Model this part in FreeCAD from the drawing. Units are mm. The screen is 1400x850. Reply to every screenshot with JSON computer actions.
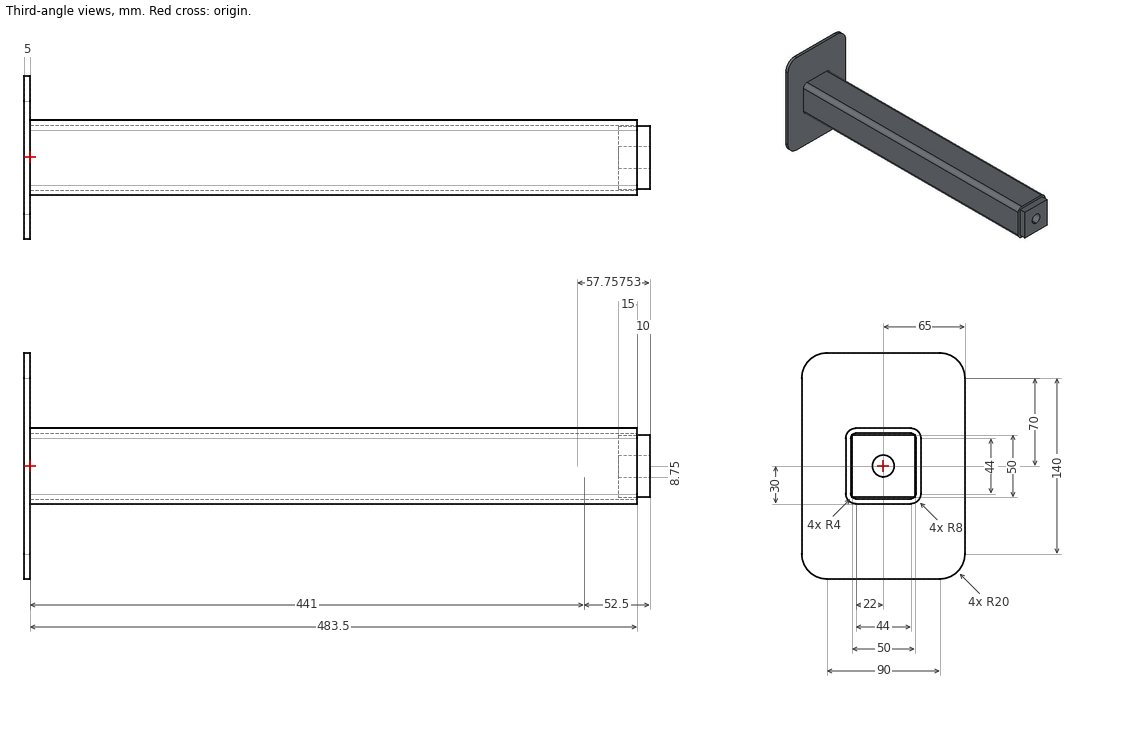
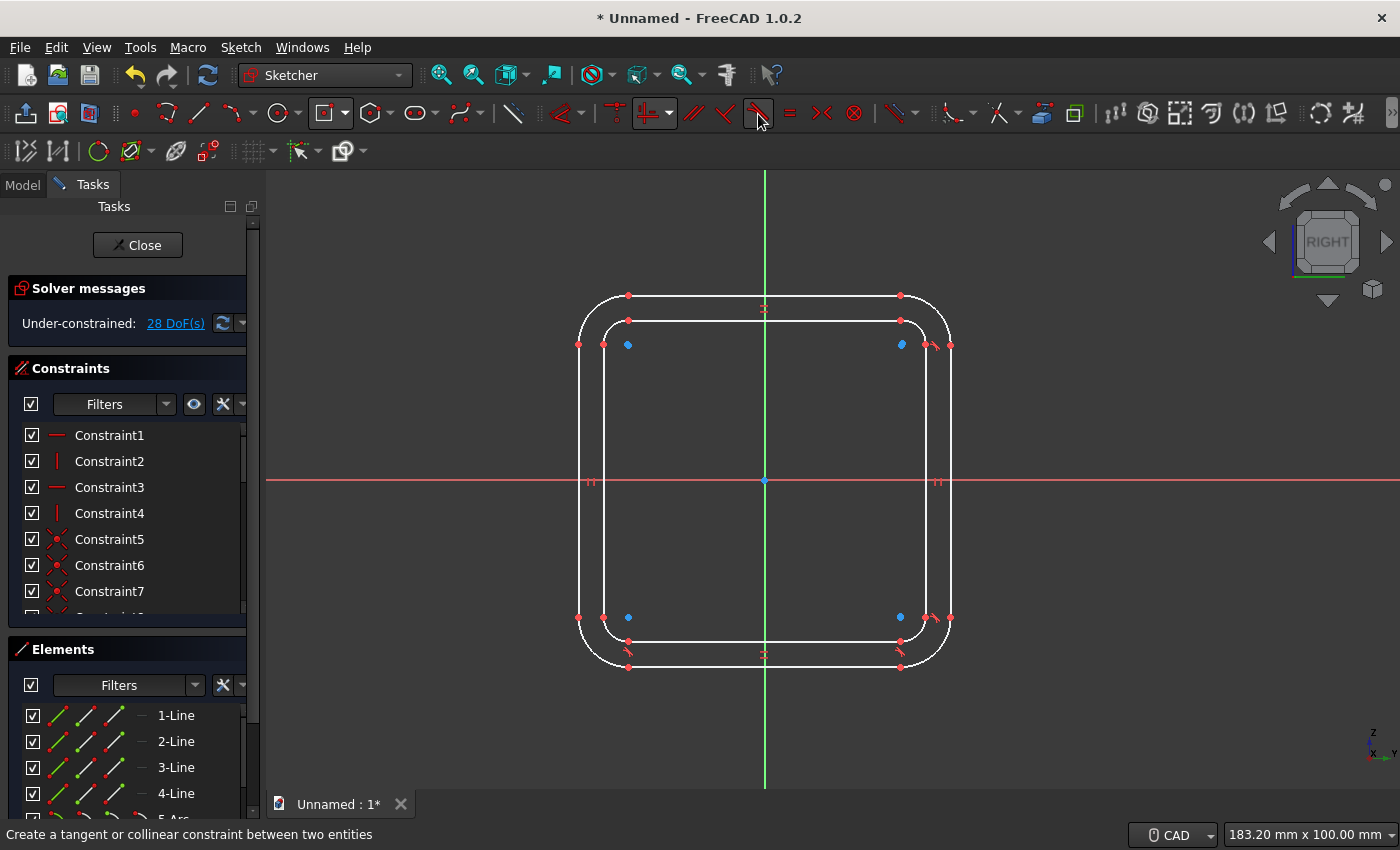
{"action": "left_click", "coordinate": [819, 296]}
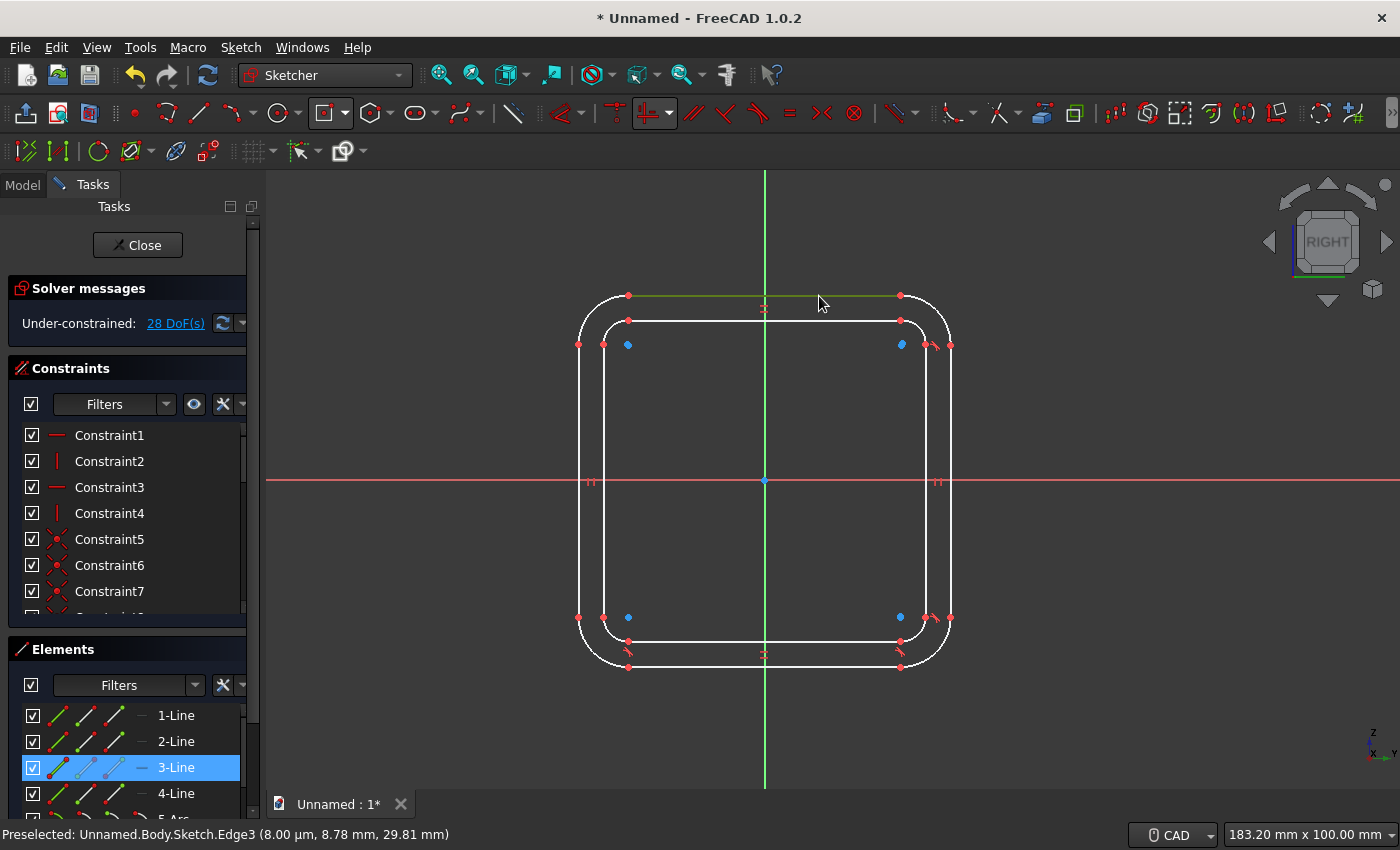
{"action": "left_click", "coordinate": [945, 322]}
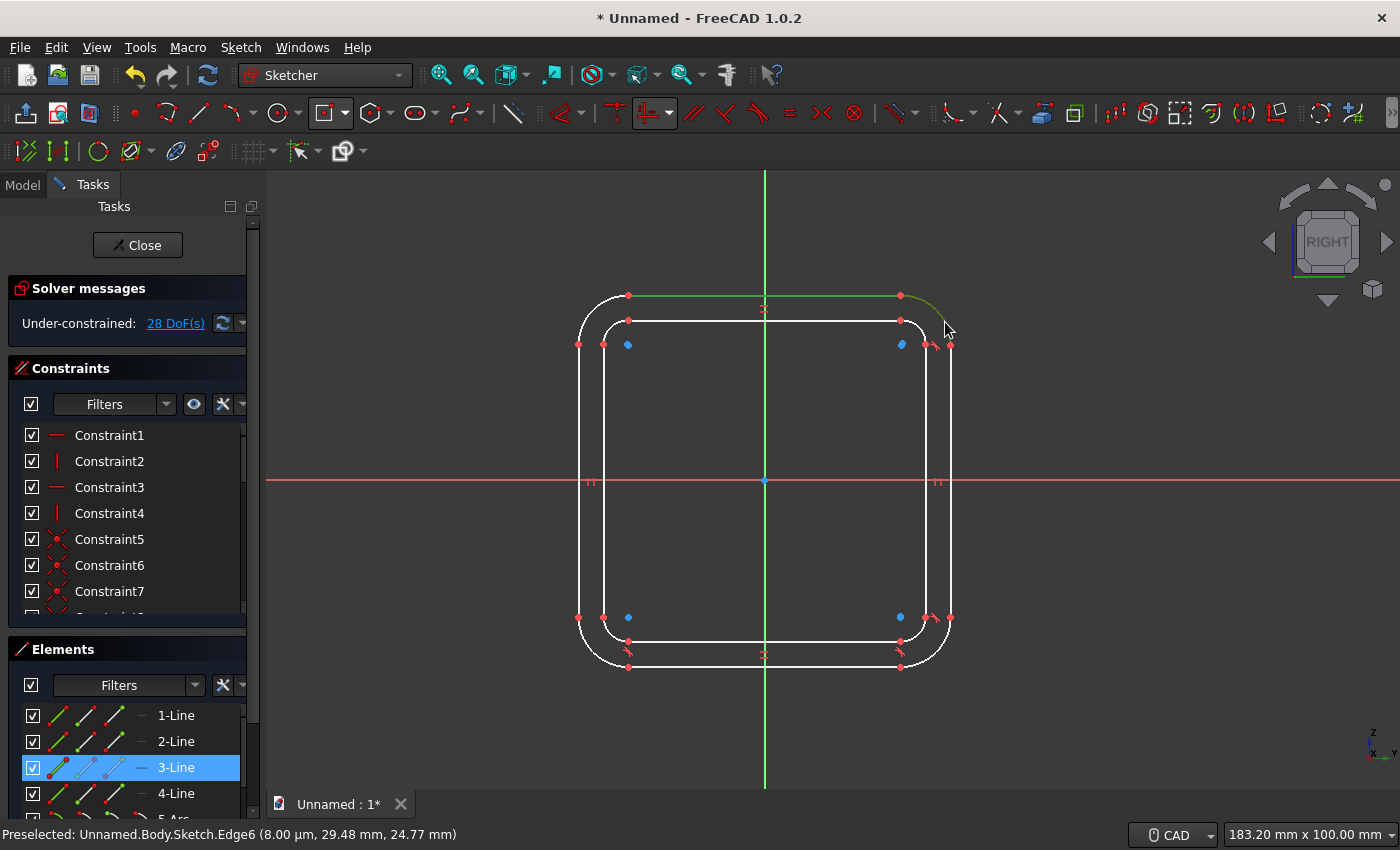
{"action": "key", "text": "t"}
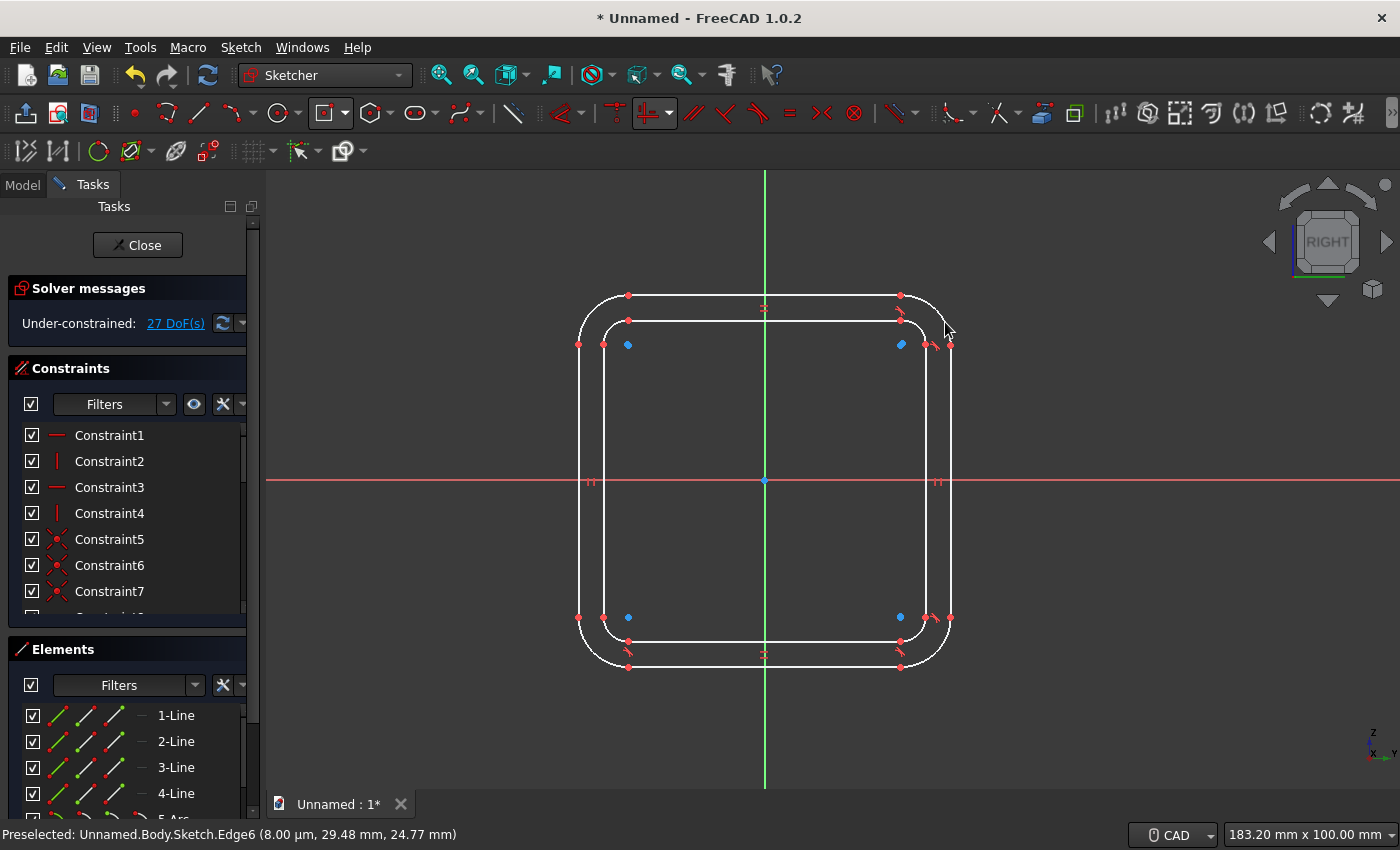
{"action": "left_click", "coordinate": [819, 295]}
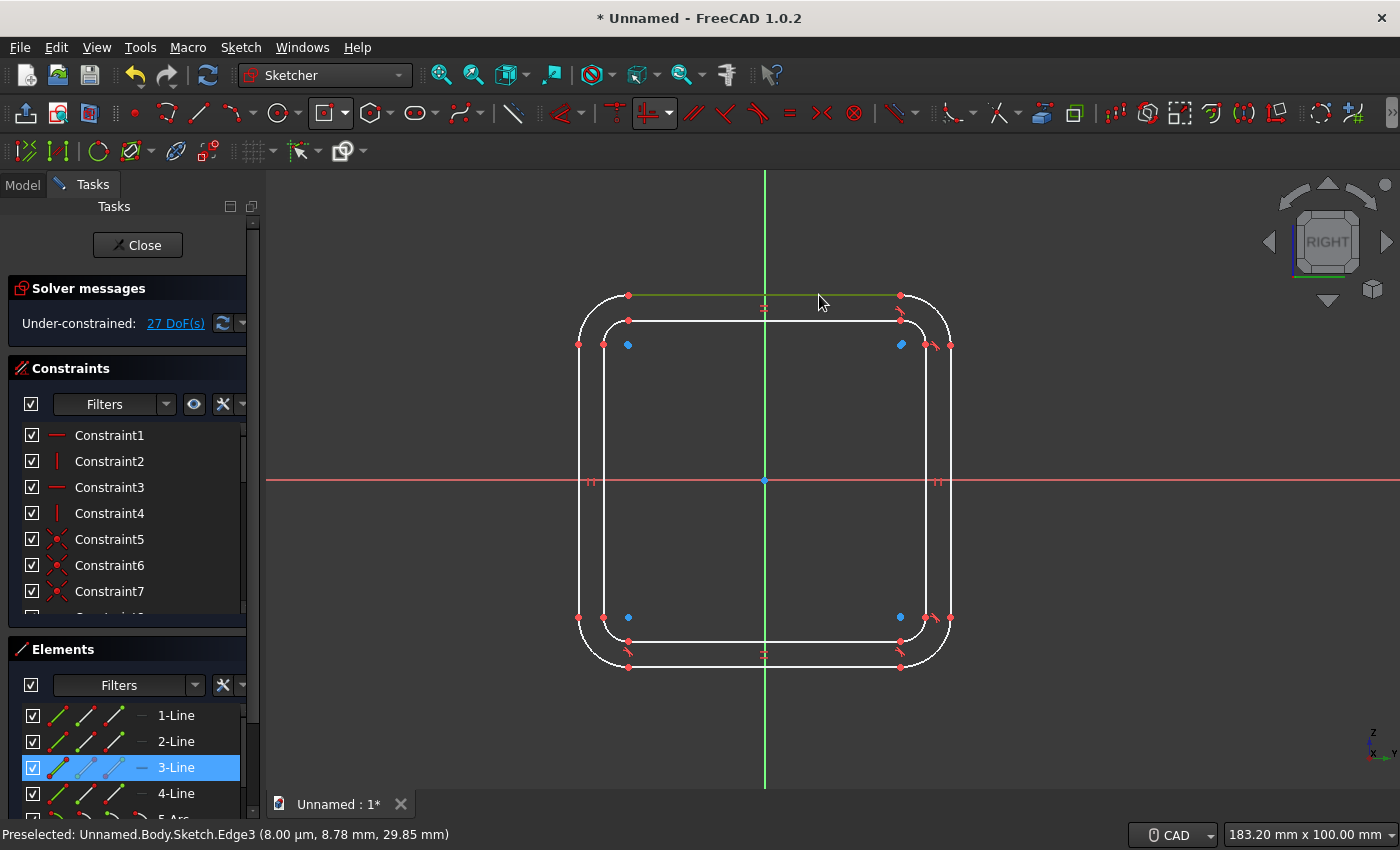
{"action": "left_click", "coordinate": [606, 301]}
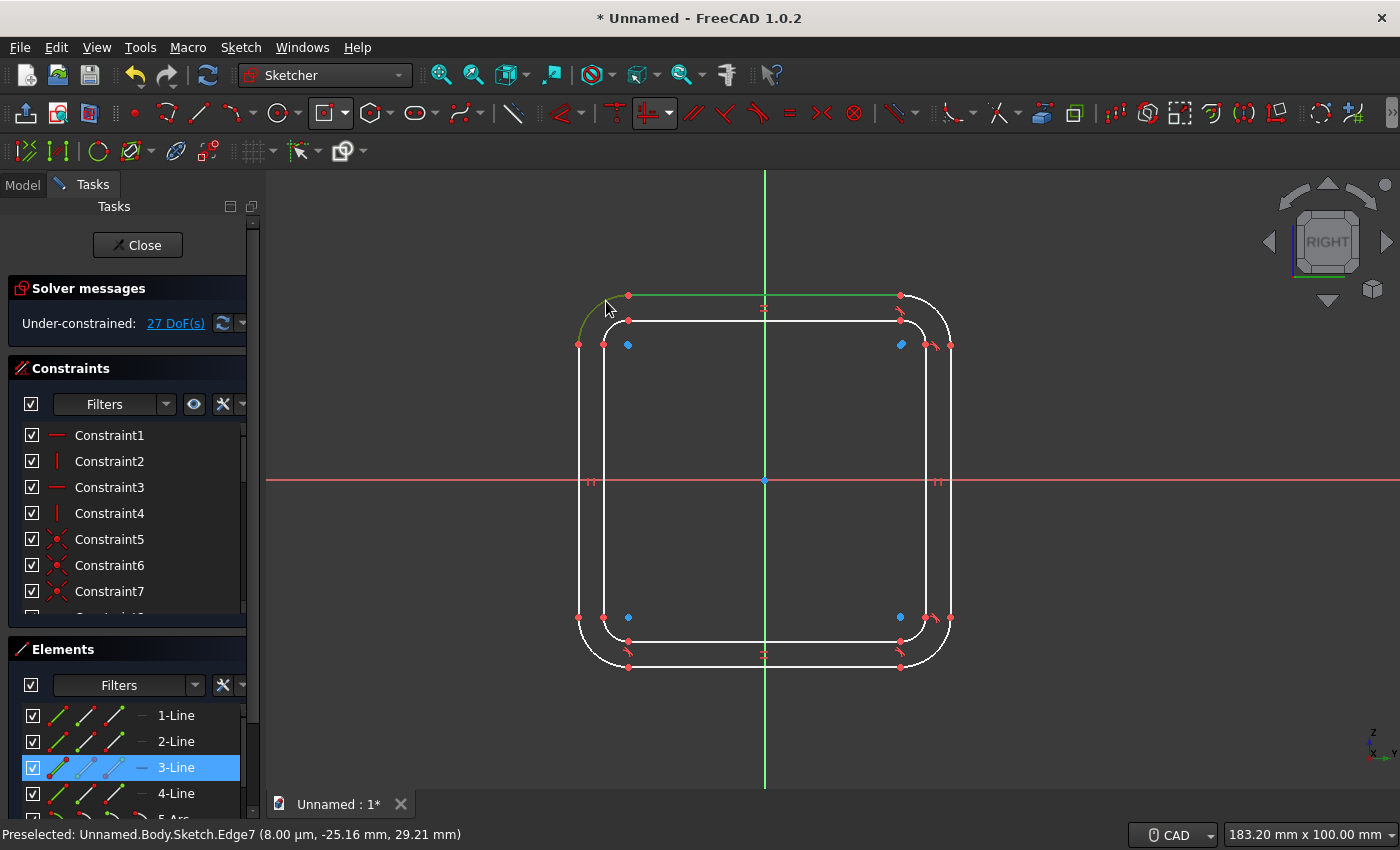
{"action": "left_click", "coordinate": [758, 114]}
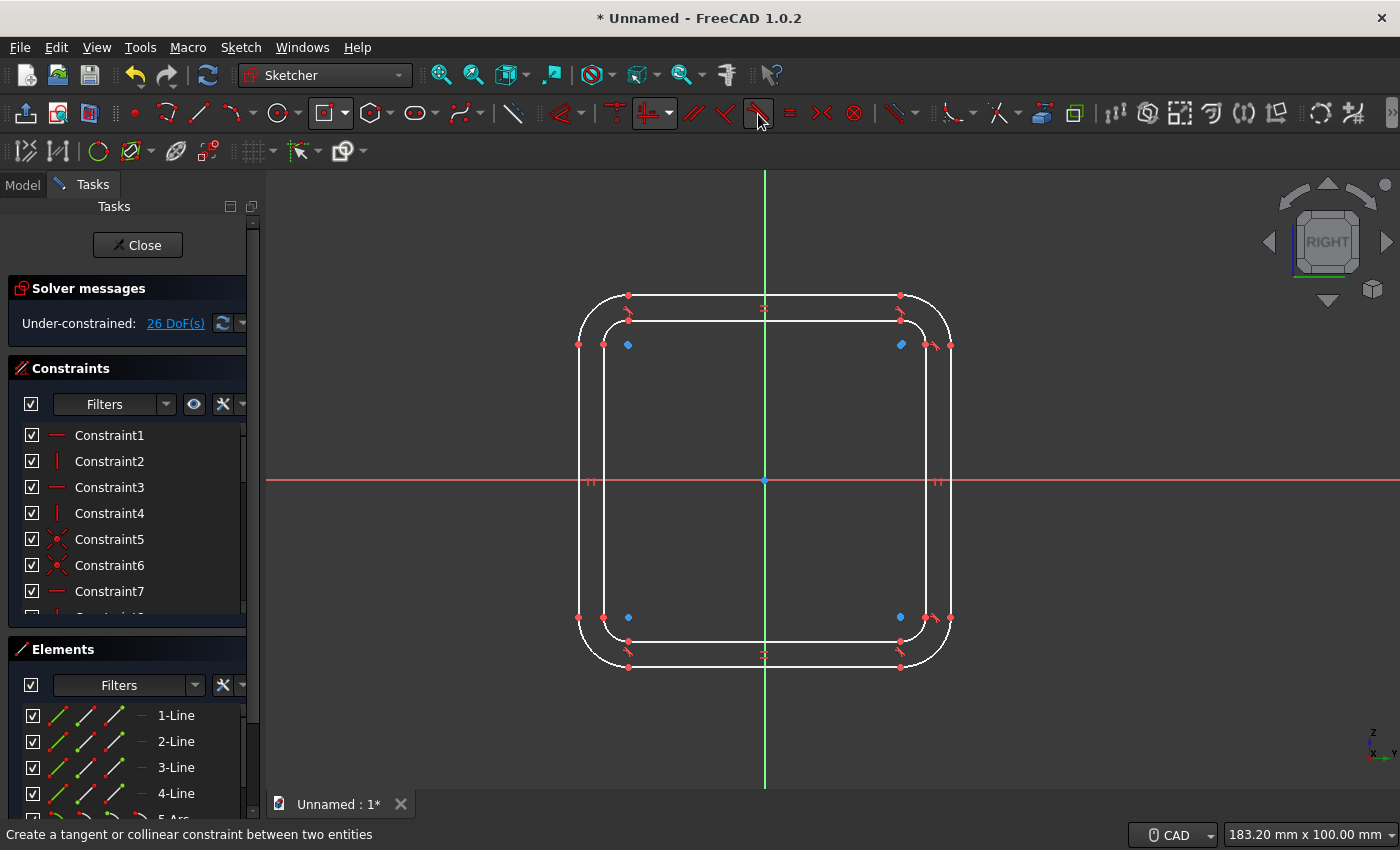
{"action": "left_click", "coordinate": [579, 426]}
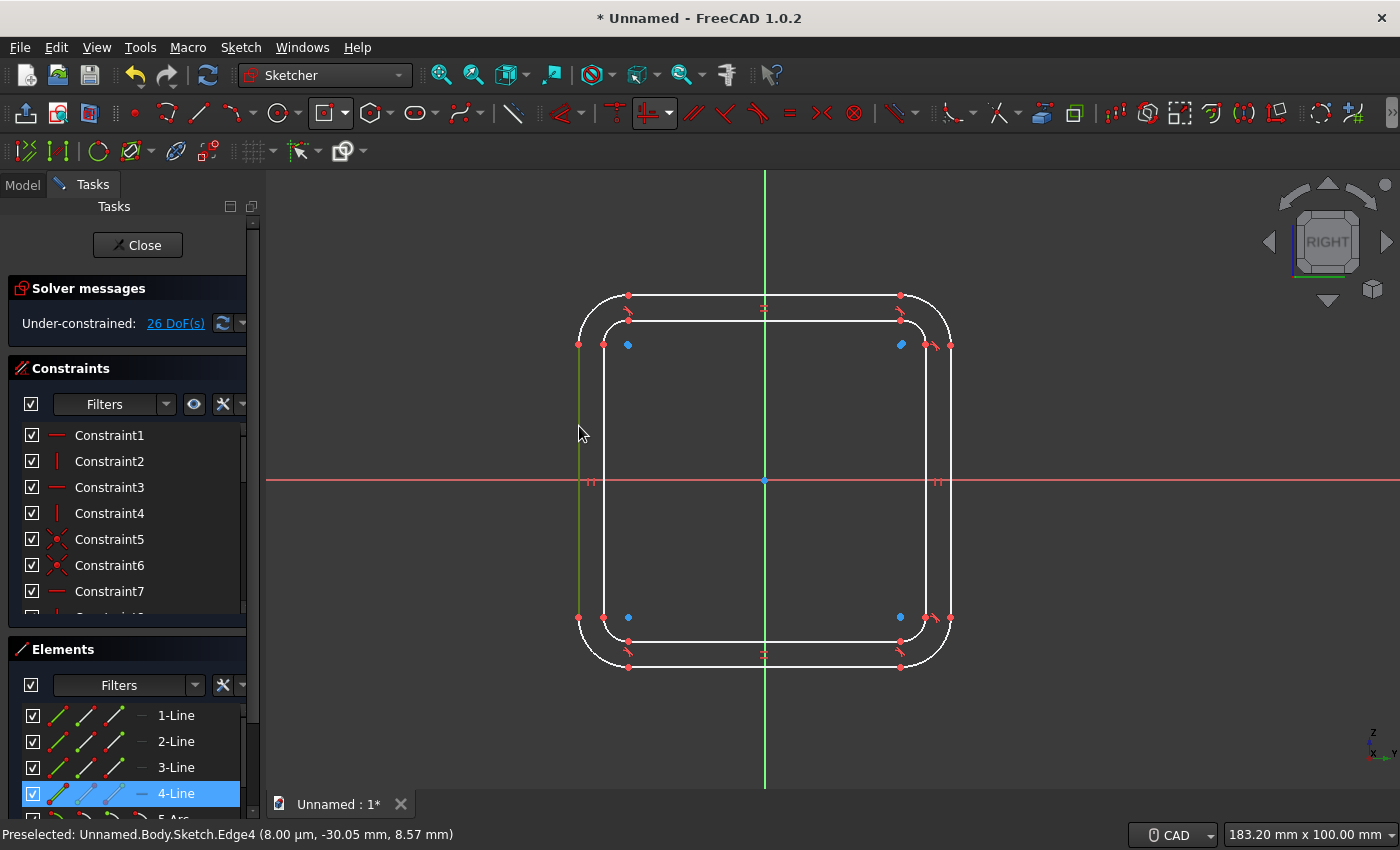
{"action": "left_click", "coordinate": [606, 300]}